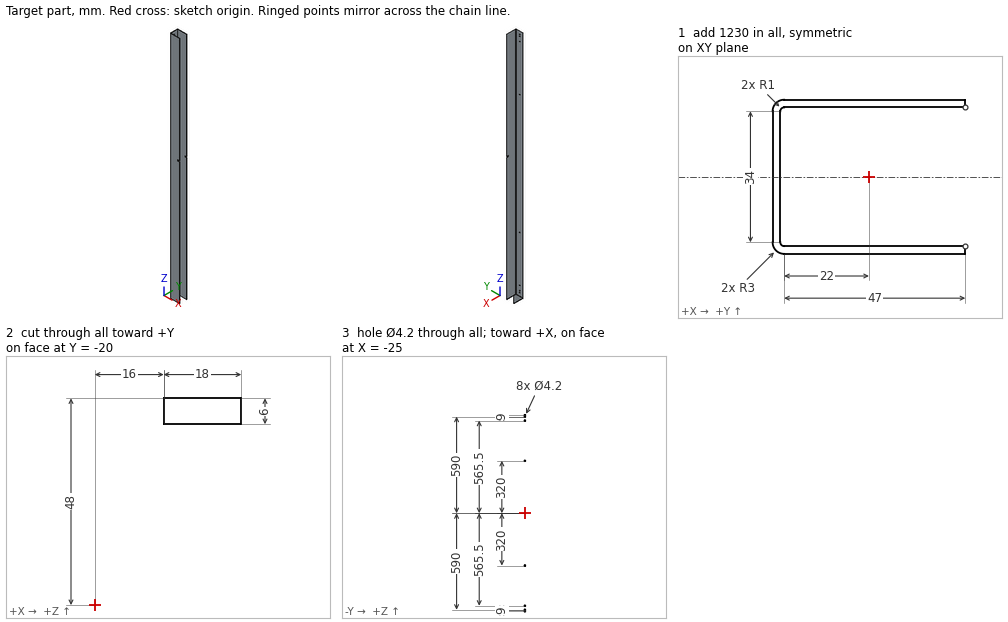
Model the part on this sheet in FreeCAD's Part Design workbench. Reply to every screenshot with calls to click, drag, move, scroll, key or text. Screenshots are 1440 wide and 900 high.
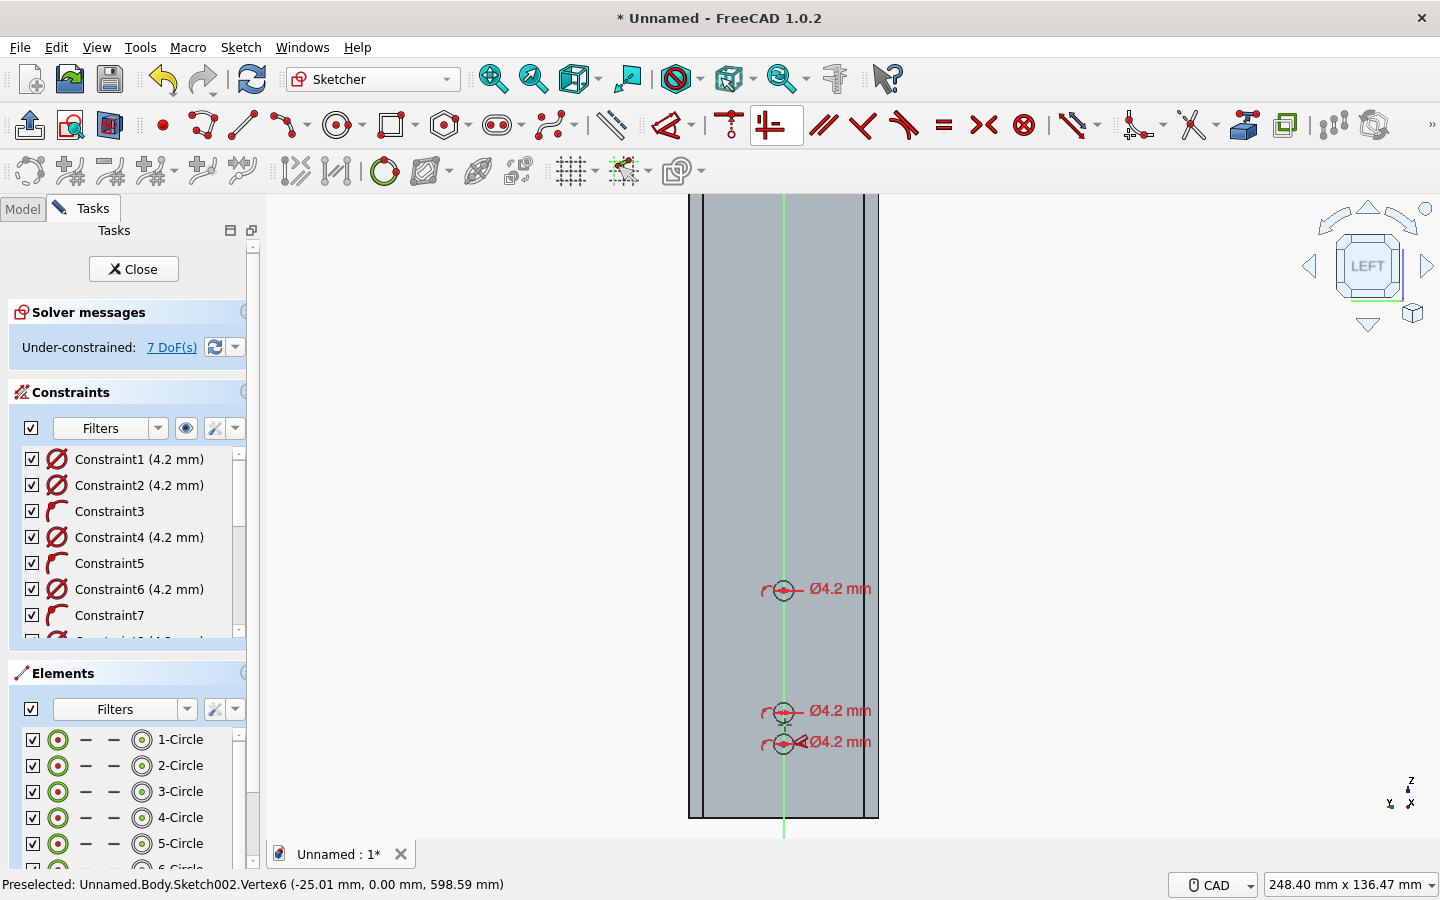
click(784, 713)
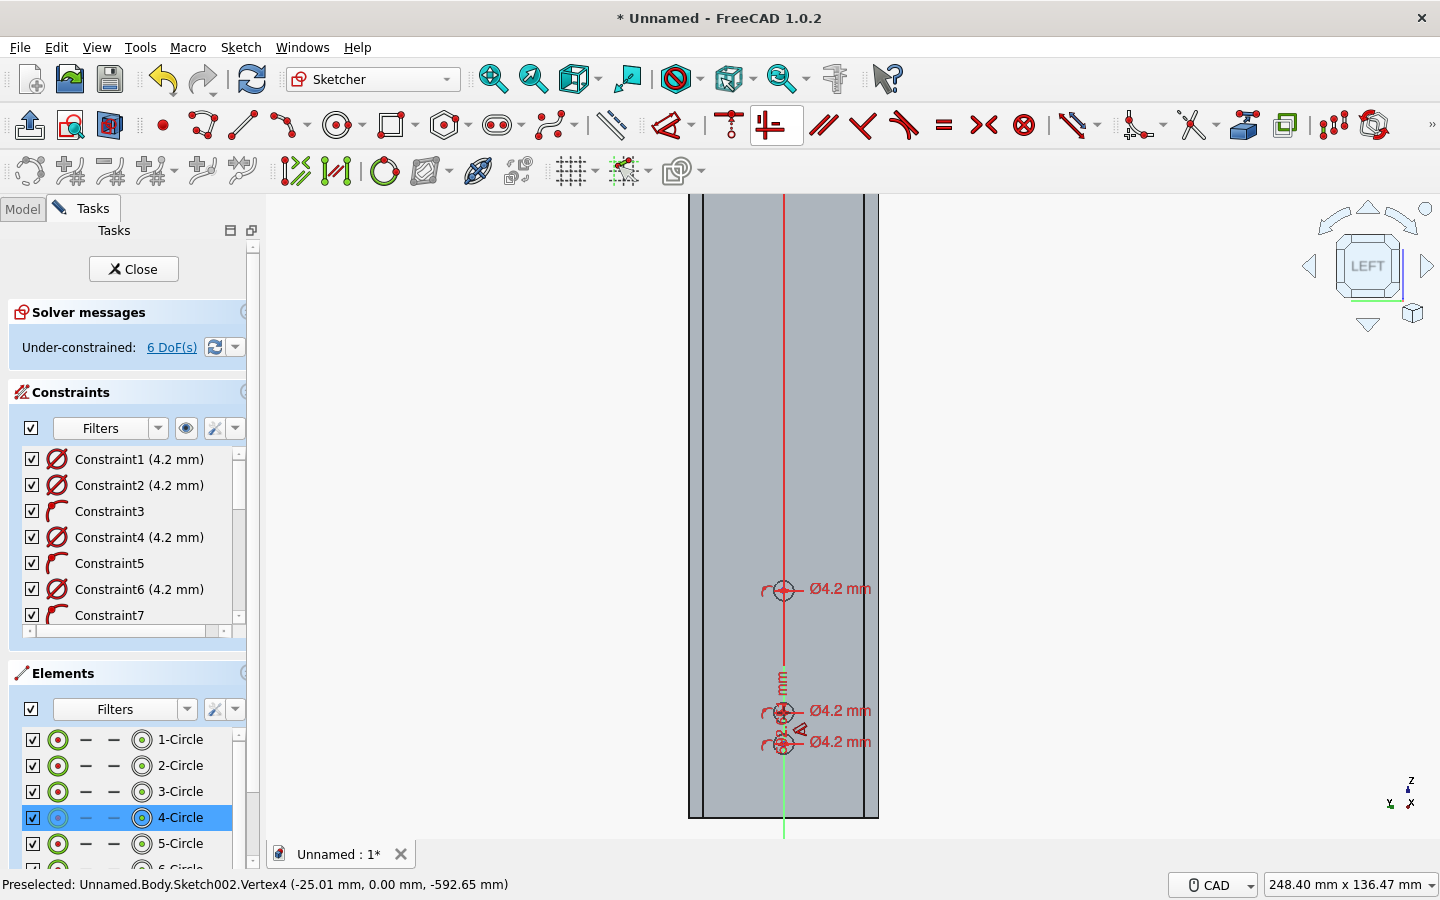
click(784, 744)
click(818, 728)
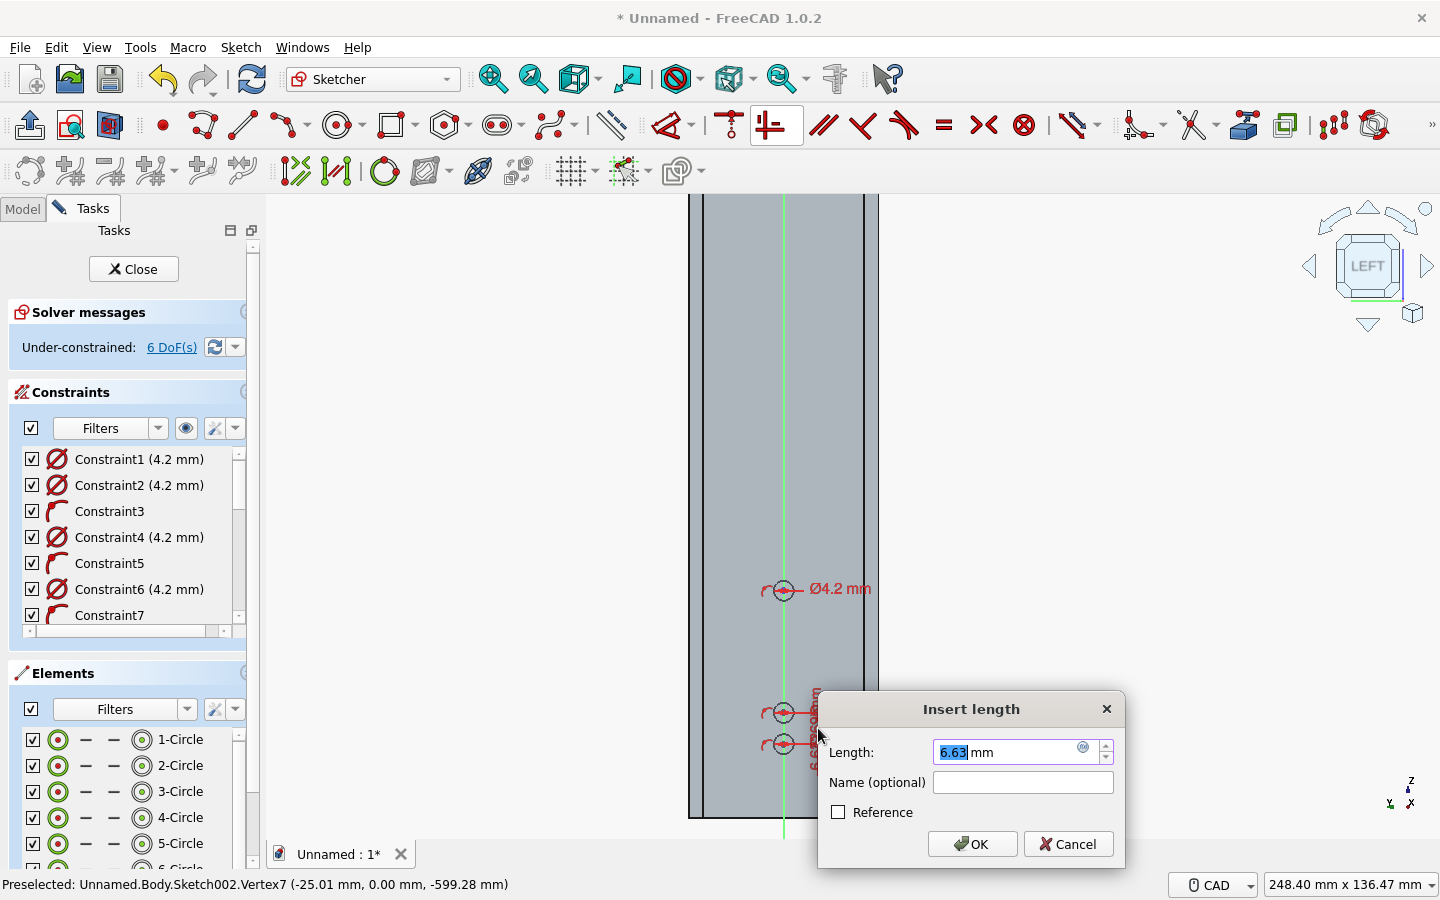
text(9)
key(Return)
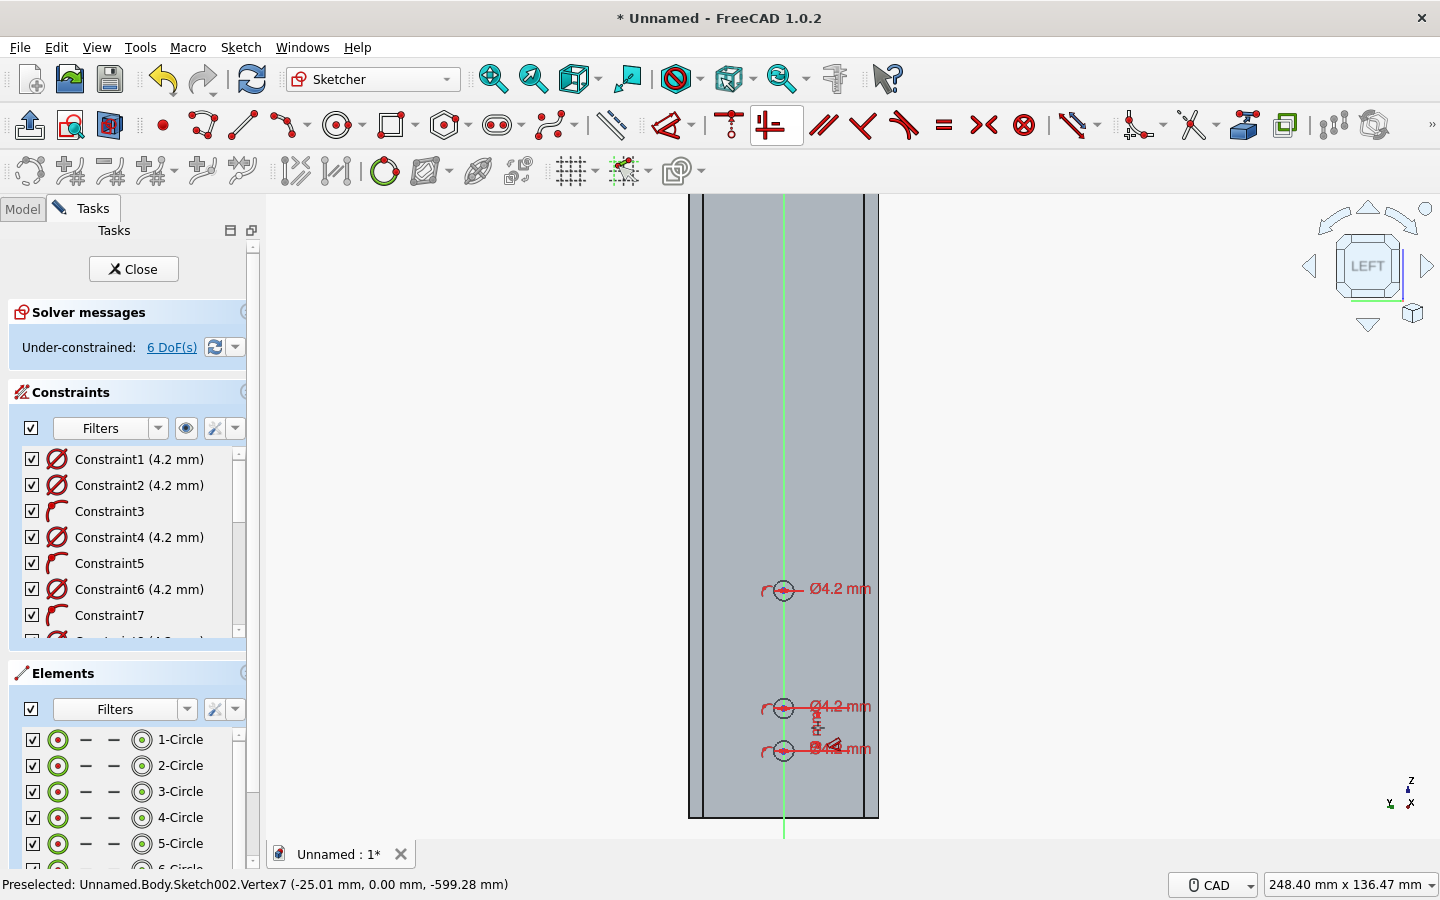
scroll(785, 725, down, 13)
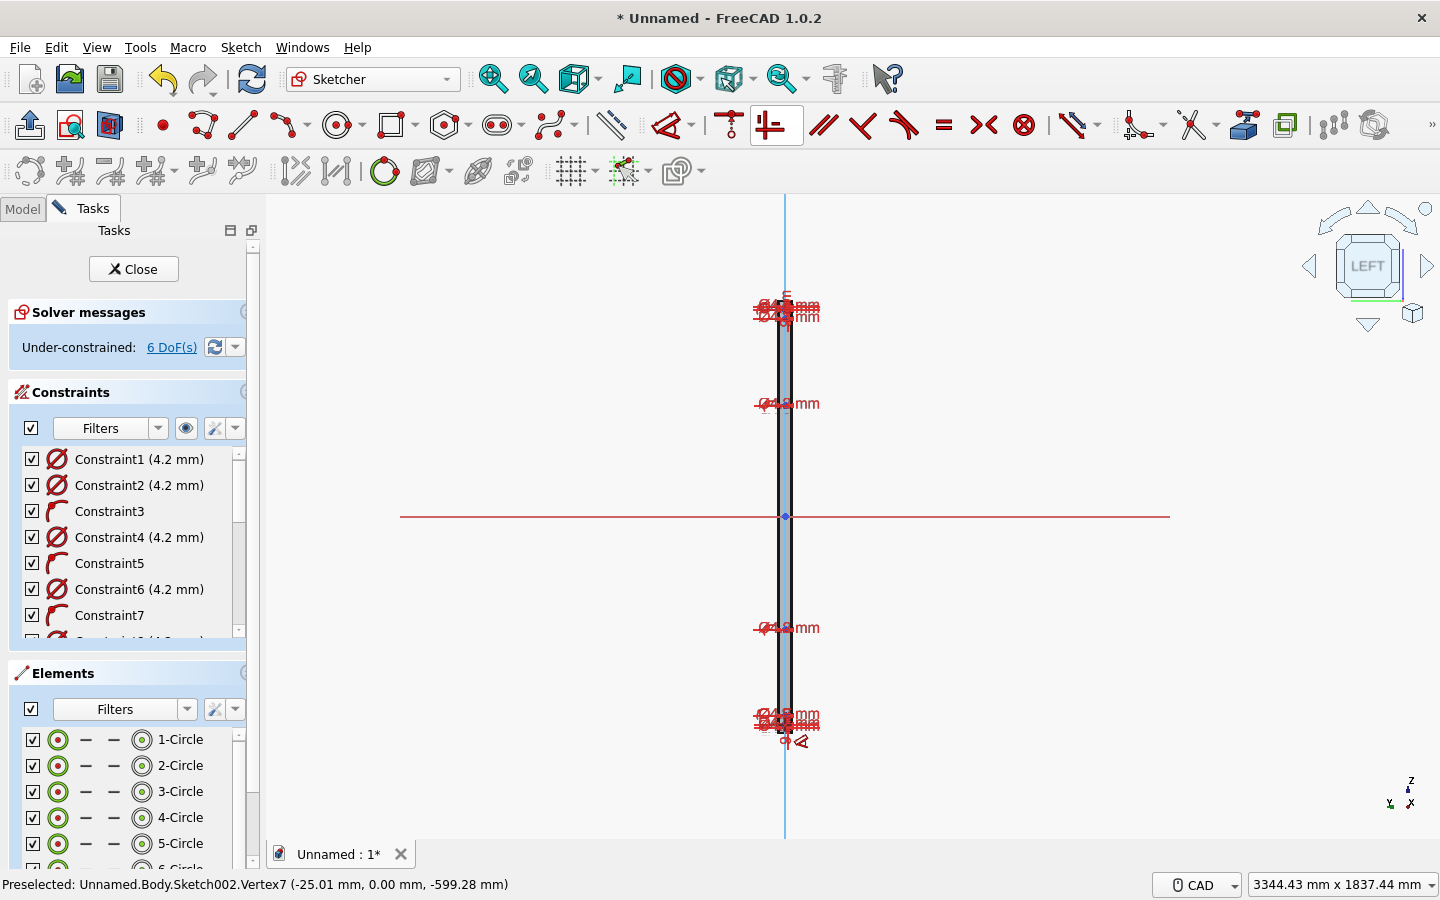
scroll(785, 310, up, 7)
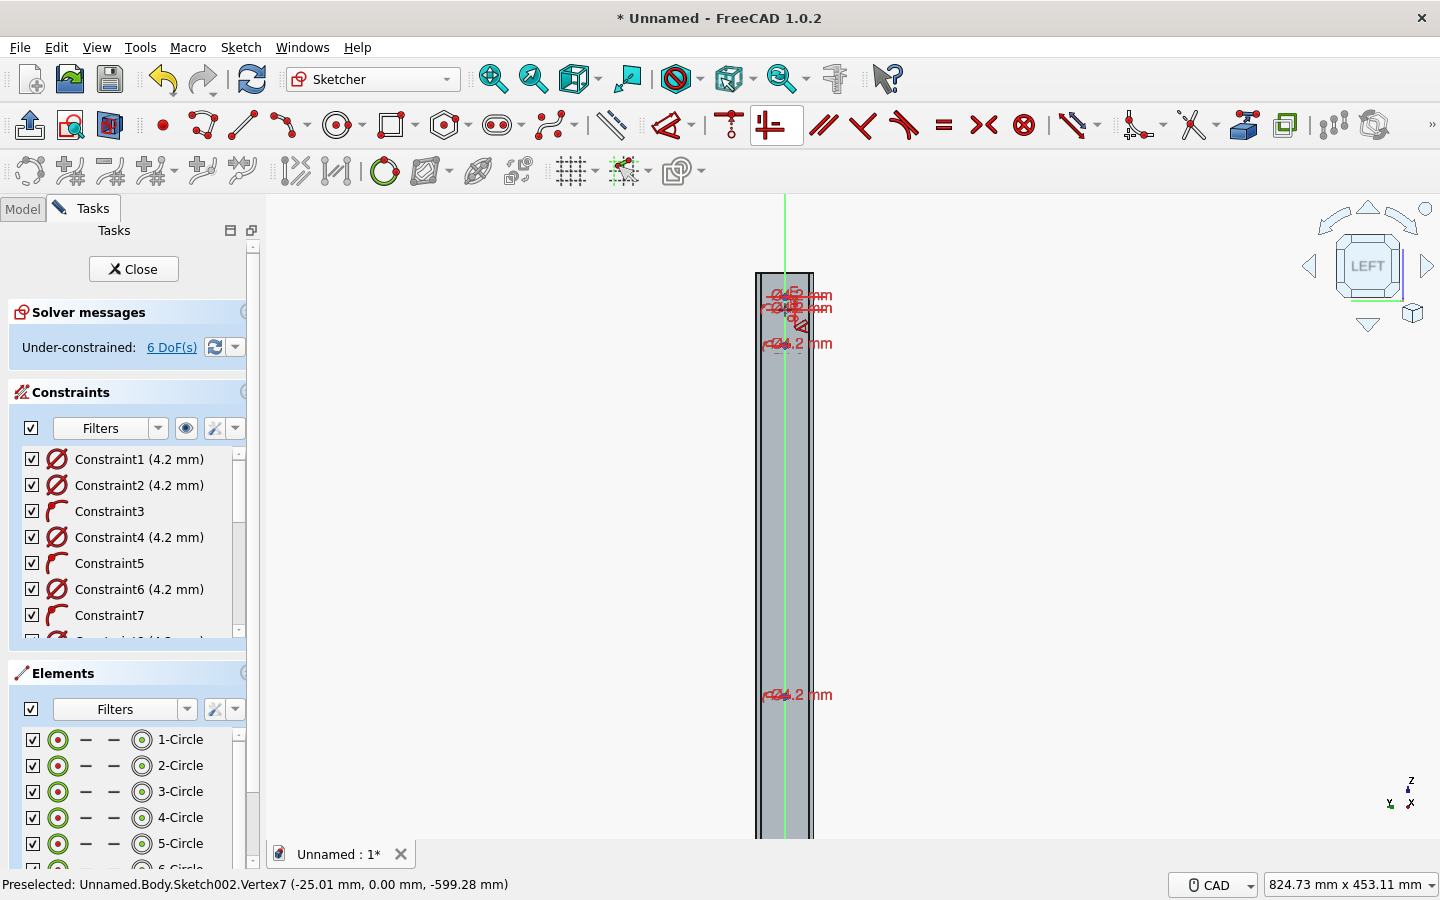
click(785, 310)
click(819, 561)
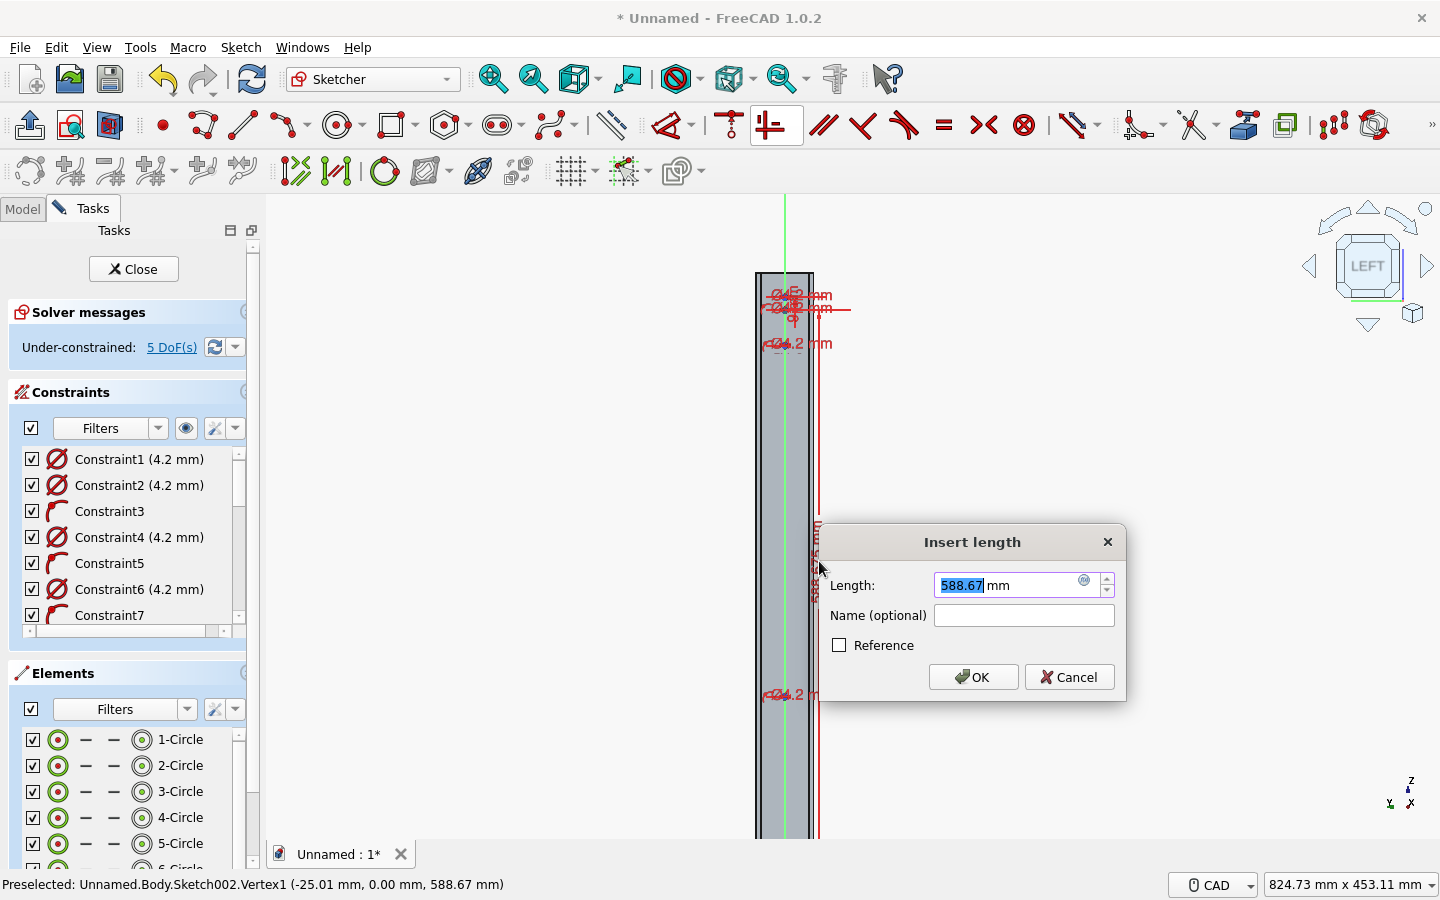
text(590)
key(Return)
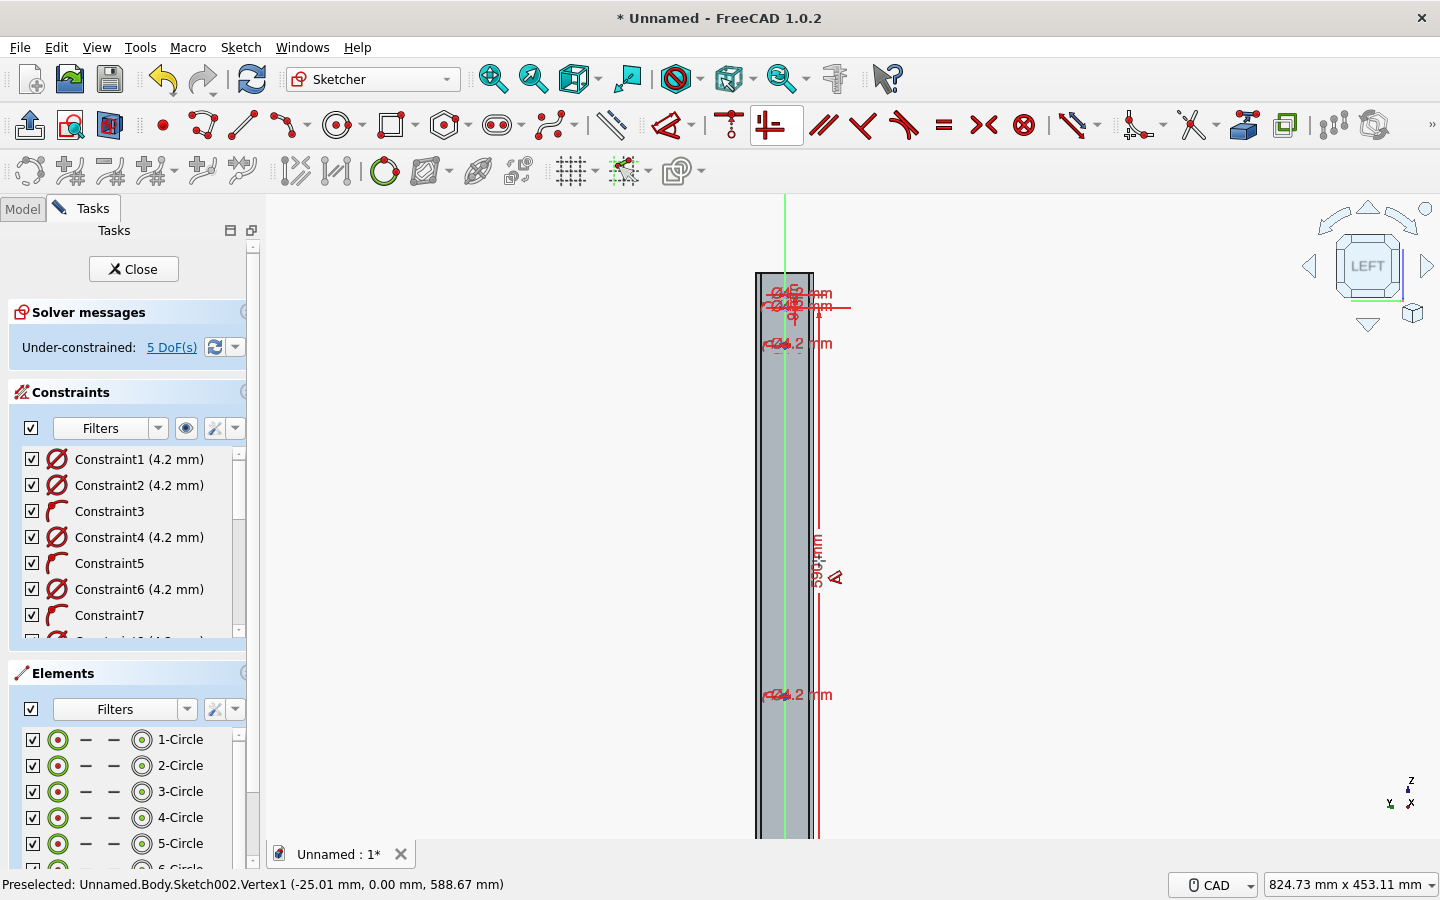
scroll(784, 310, down, 7)